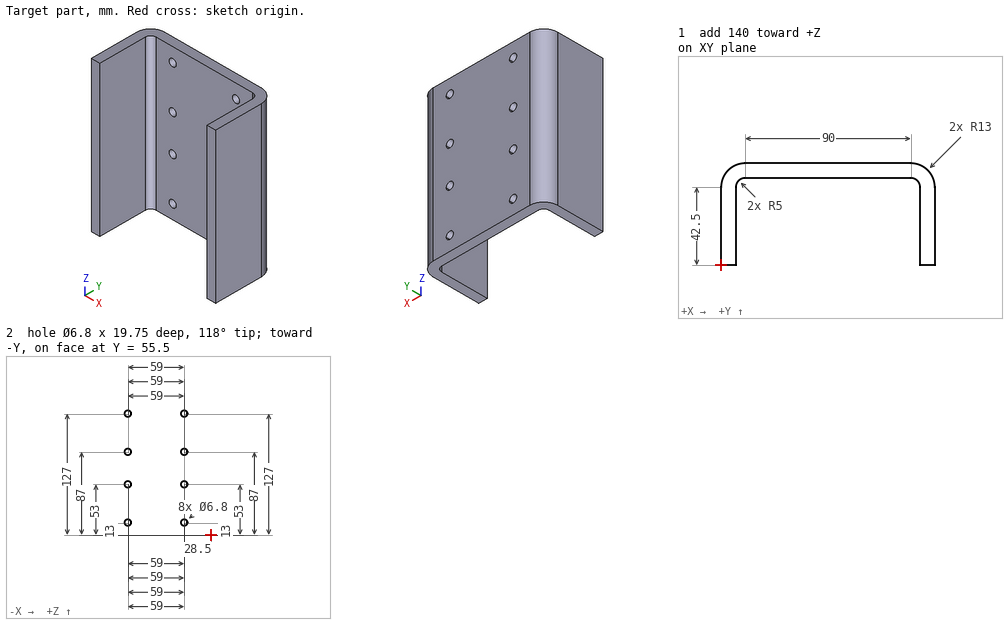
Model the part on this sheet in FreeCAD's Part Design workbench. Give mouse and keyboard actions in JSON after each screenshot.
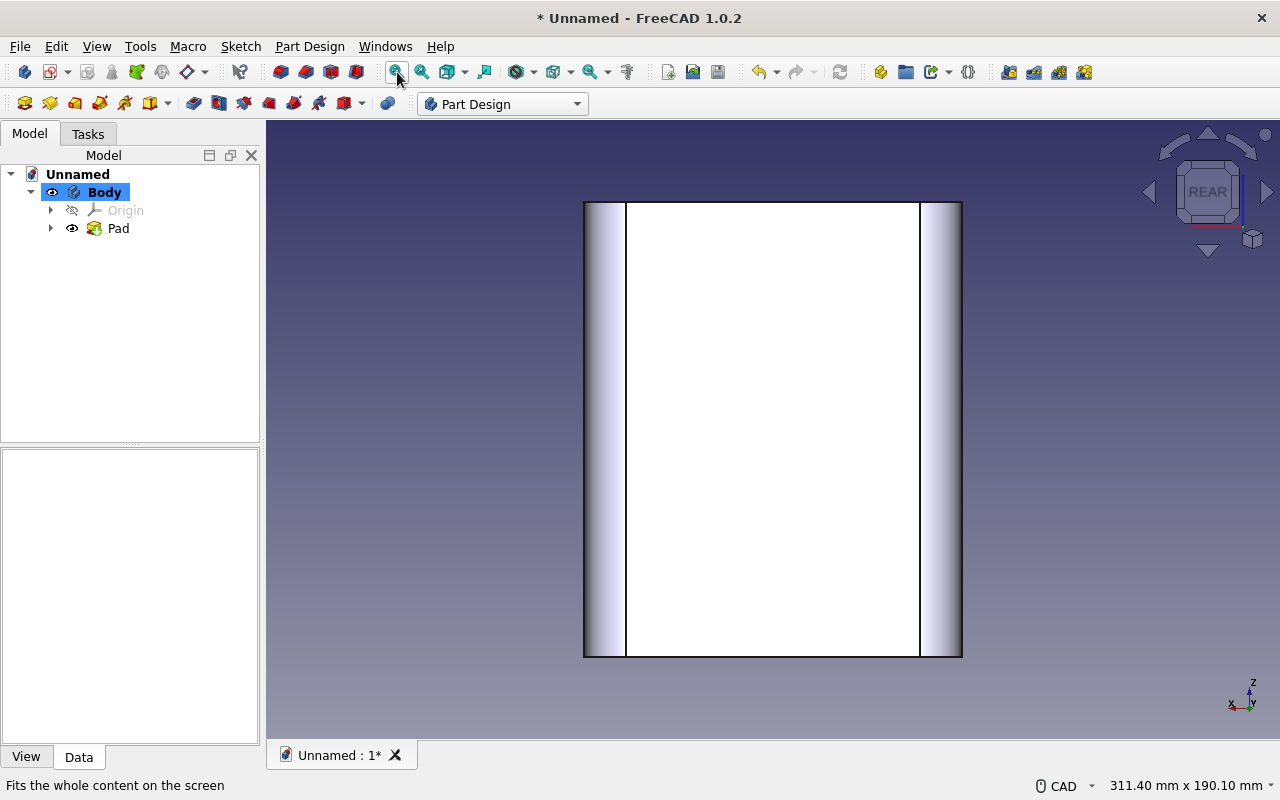
{"action": "left_click", "coordinate": [773, 363]}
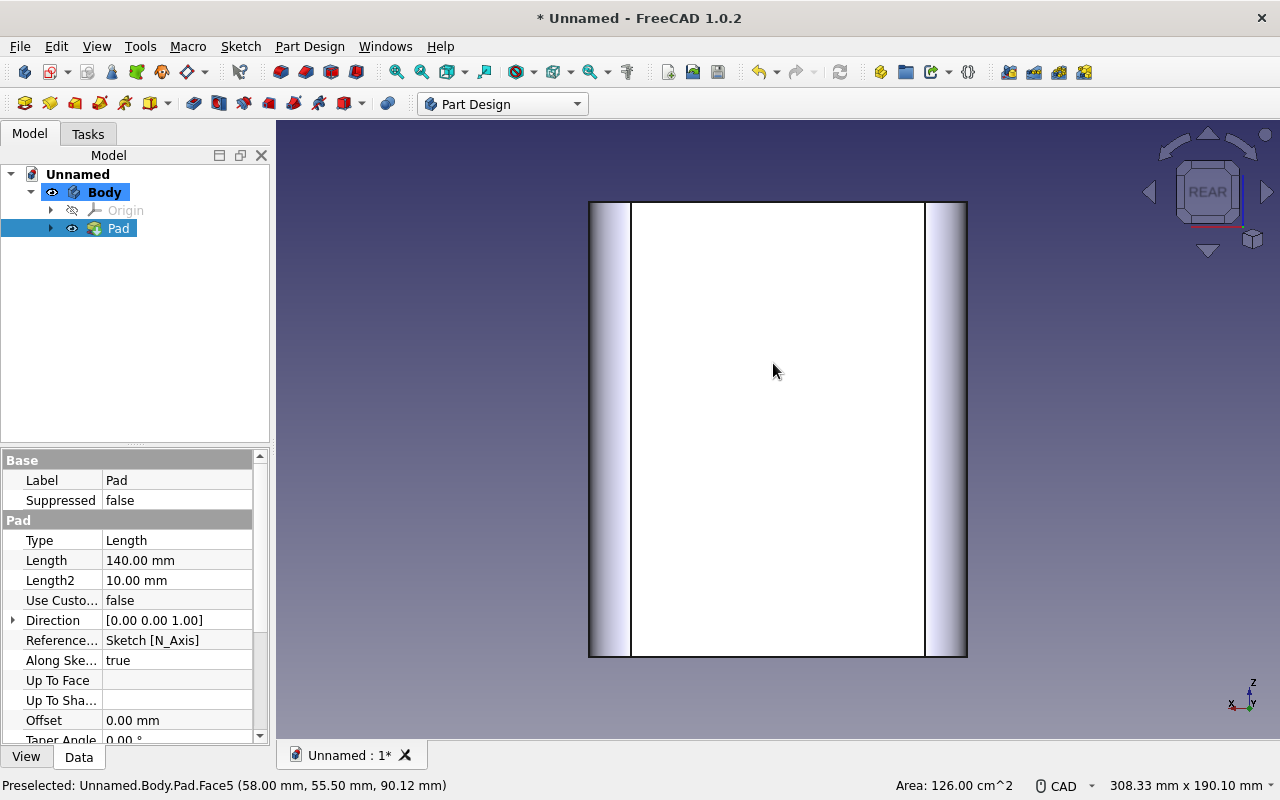
{"action": "left_click", "coordinate": [50, 72]}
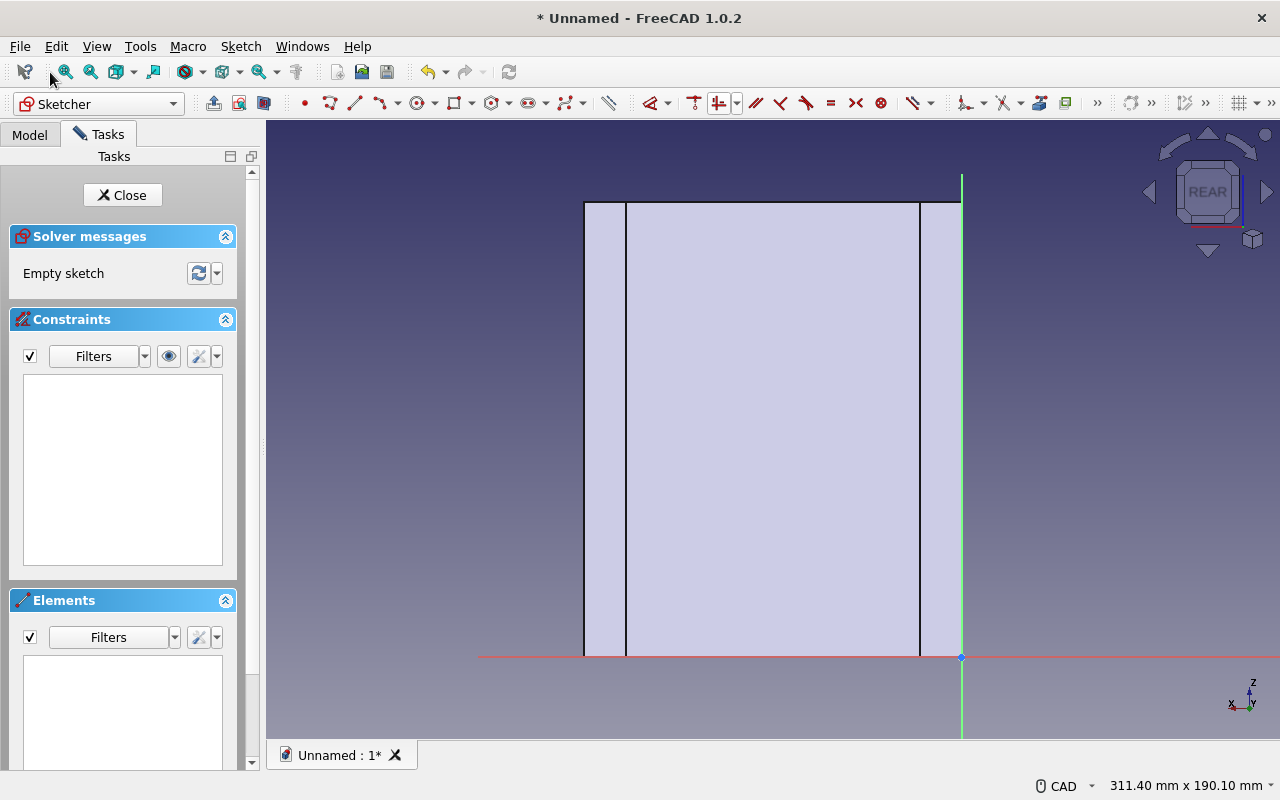
{"action": "key", "text": "g c"}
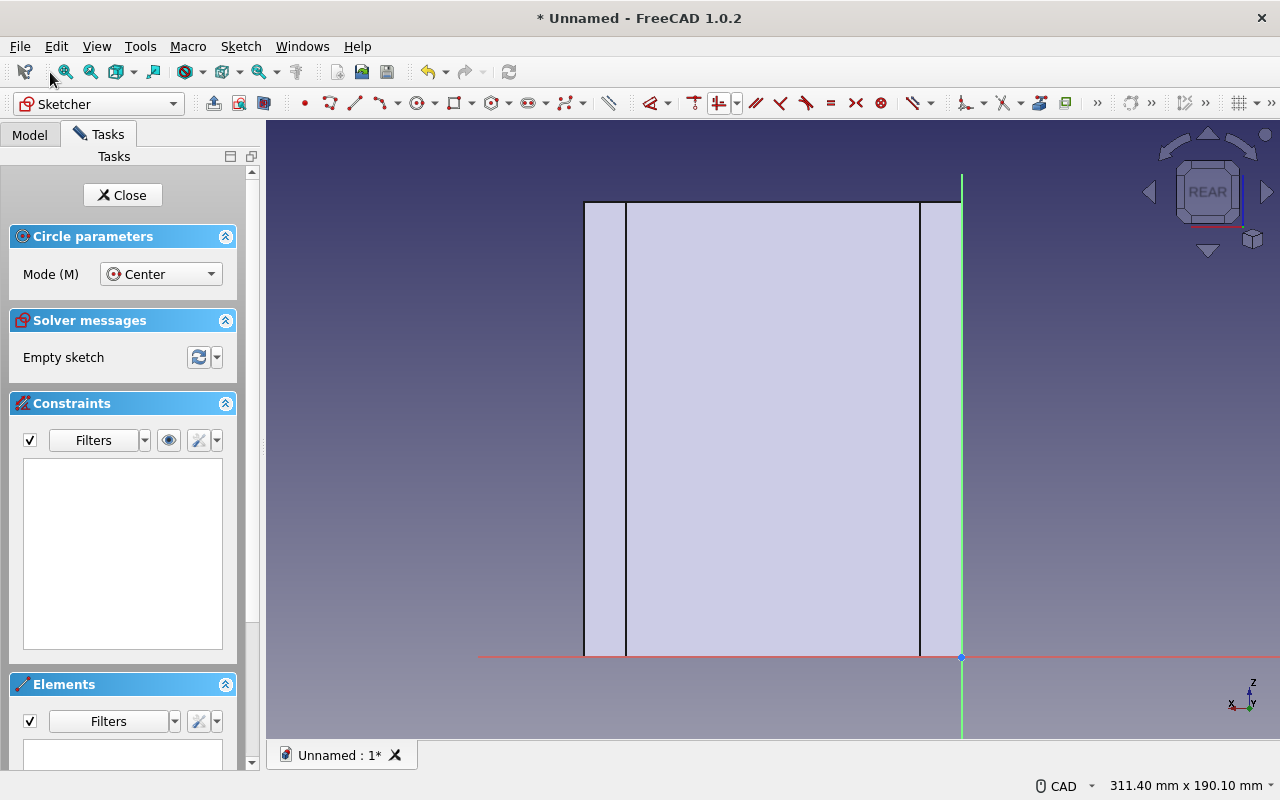
{"action": "scroll", "coordinate": [869, 615], "scroll_direction": "up", "scroll_amount": 4}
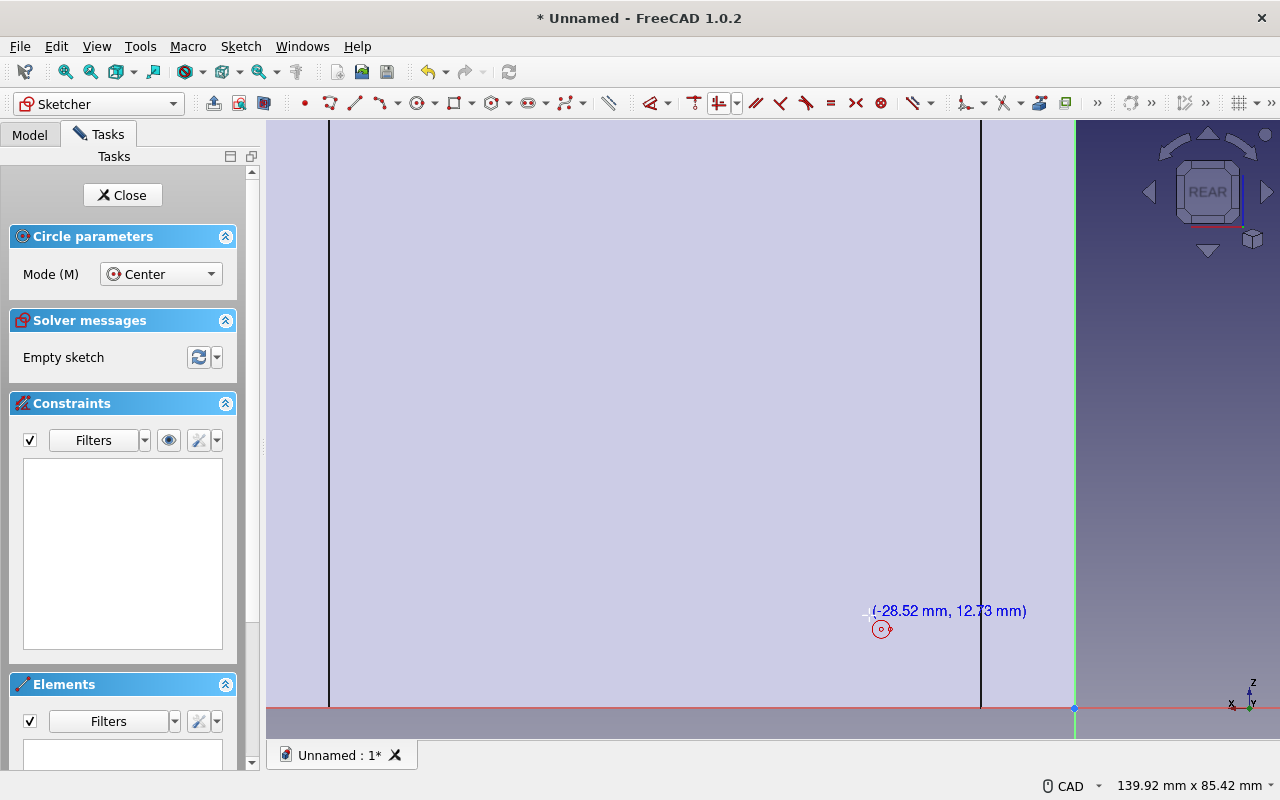
{"action": "left_click", "coordinate": [868, 614]}
{"action": "mouse_move", "coordinate": [886, 597]}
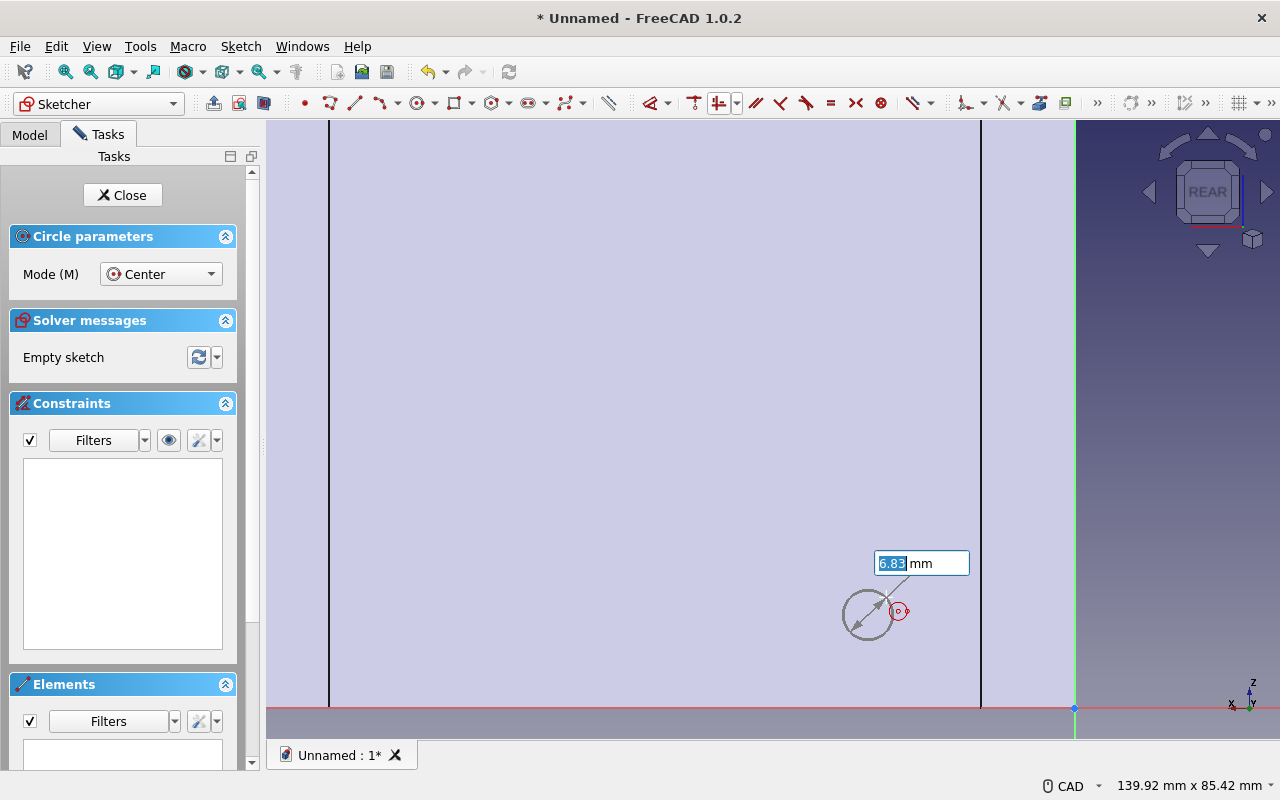
{"action": "type", "text": "6.8"}
{"action": "key", "text": "Return"}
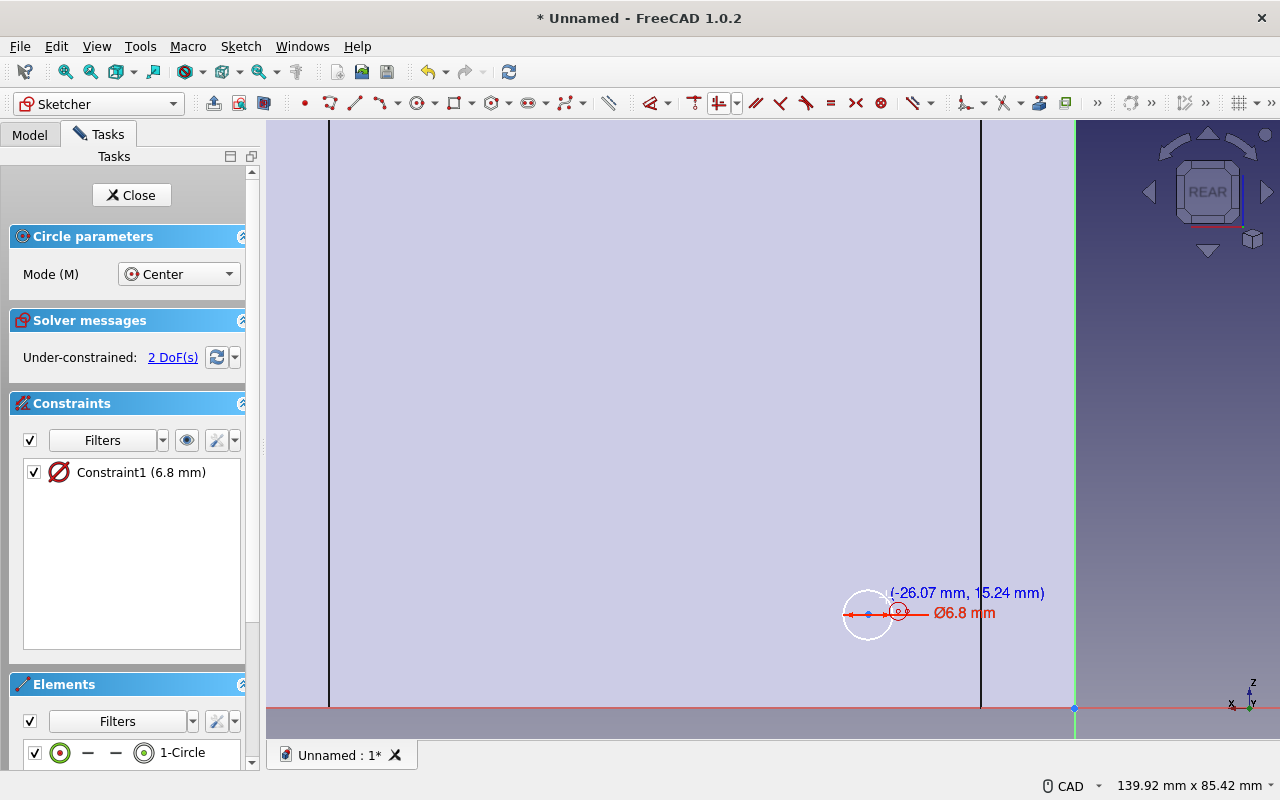
{"action": "left_click", "coordinate": [441, 614]}
{"action": "mouse_move", "coordinate": [458, 597]}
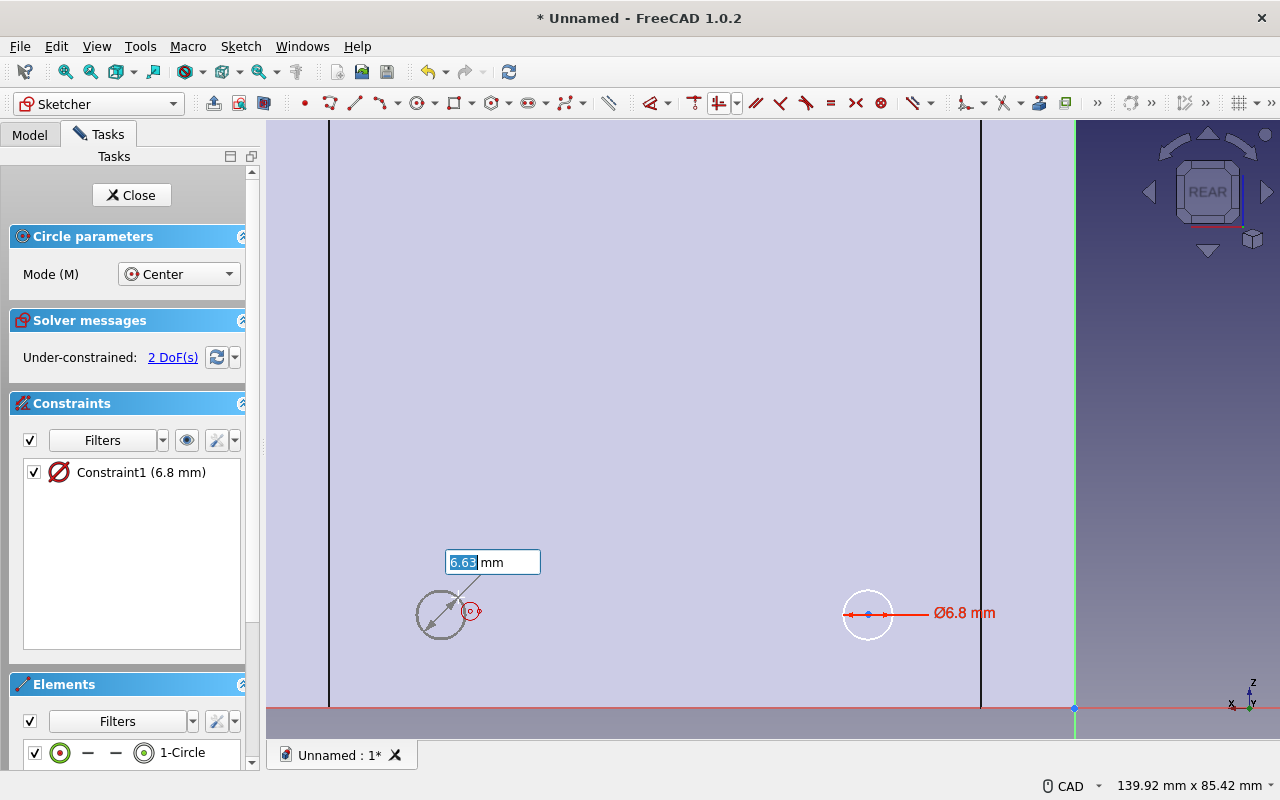
{"action": "type", "text": "6.8"}
{"action": "key", "text": "Return"}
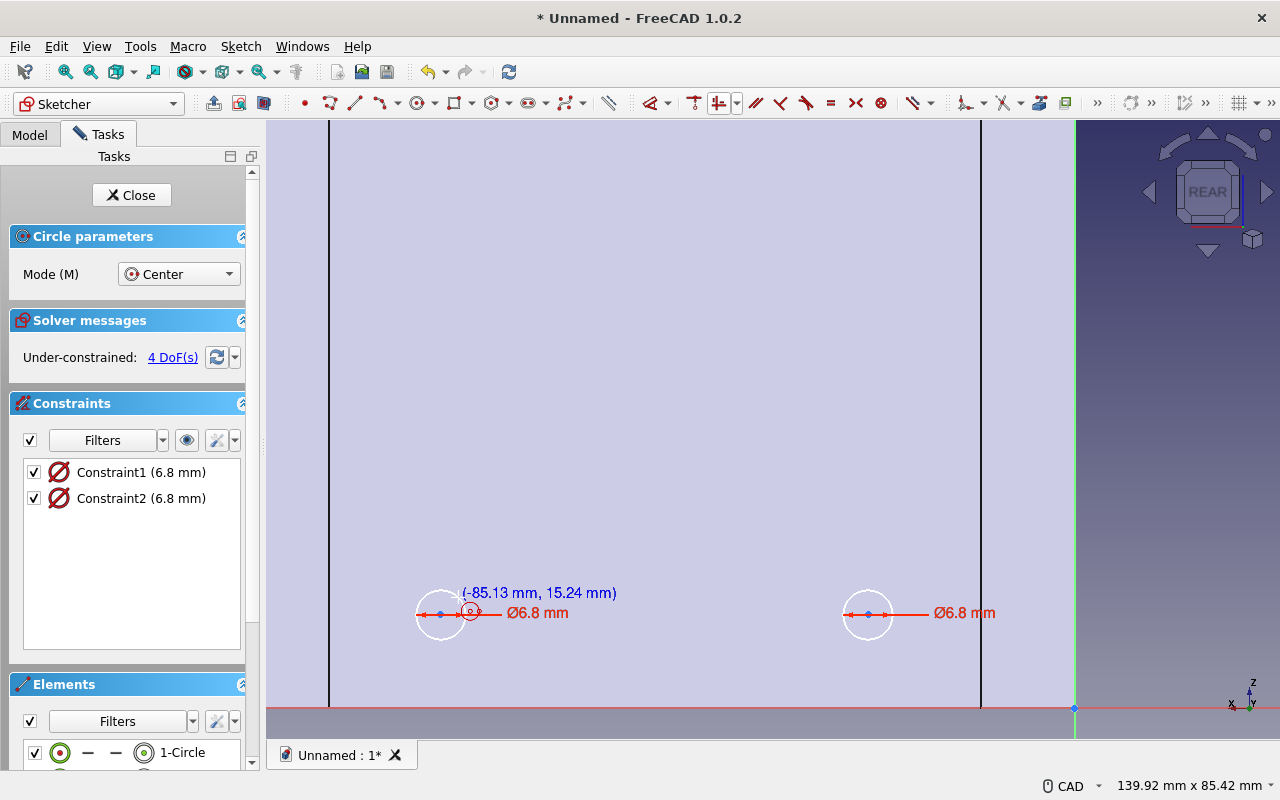
{"action": "left_click", "coordinate": [441, 324]}
{"action": "mouse_move", "coordinate": [458, 307]}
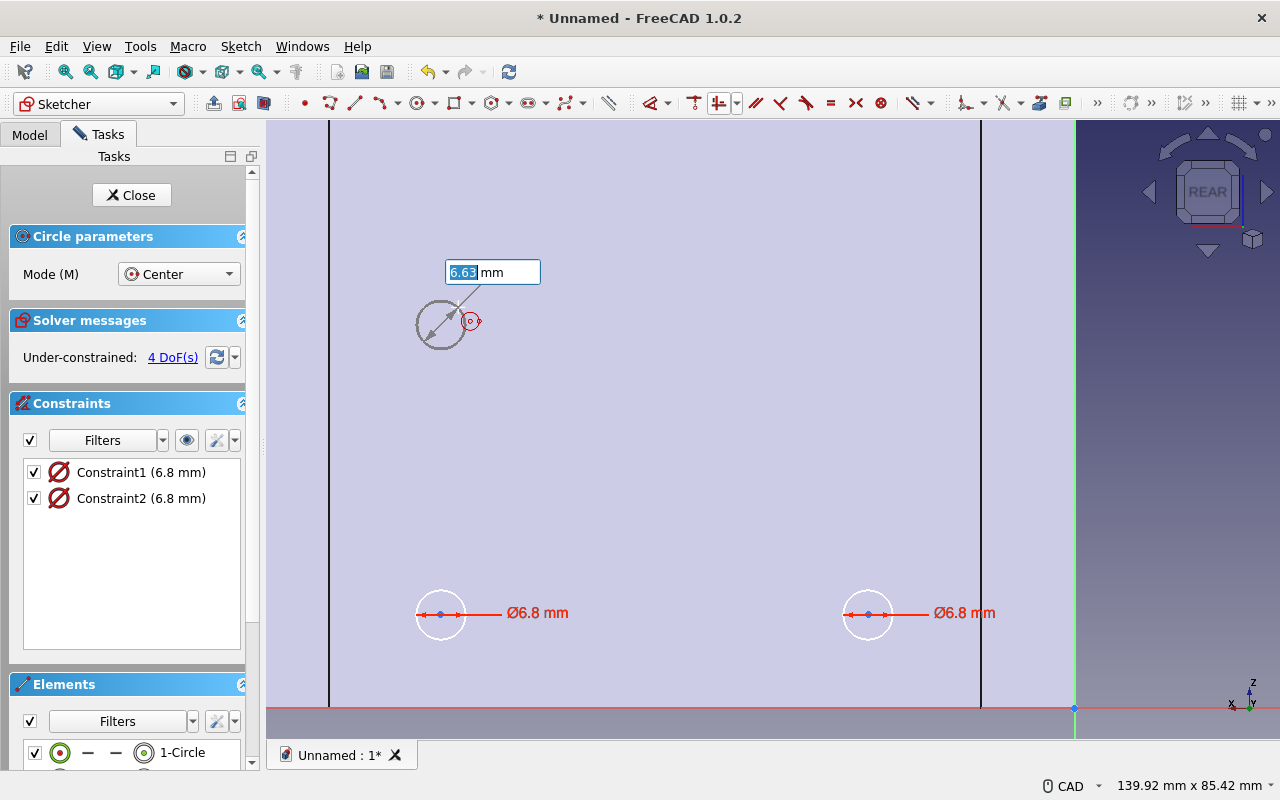
{"action": "type", "text": "6.8"}
{"action": "key", "text": "Return"}